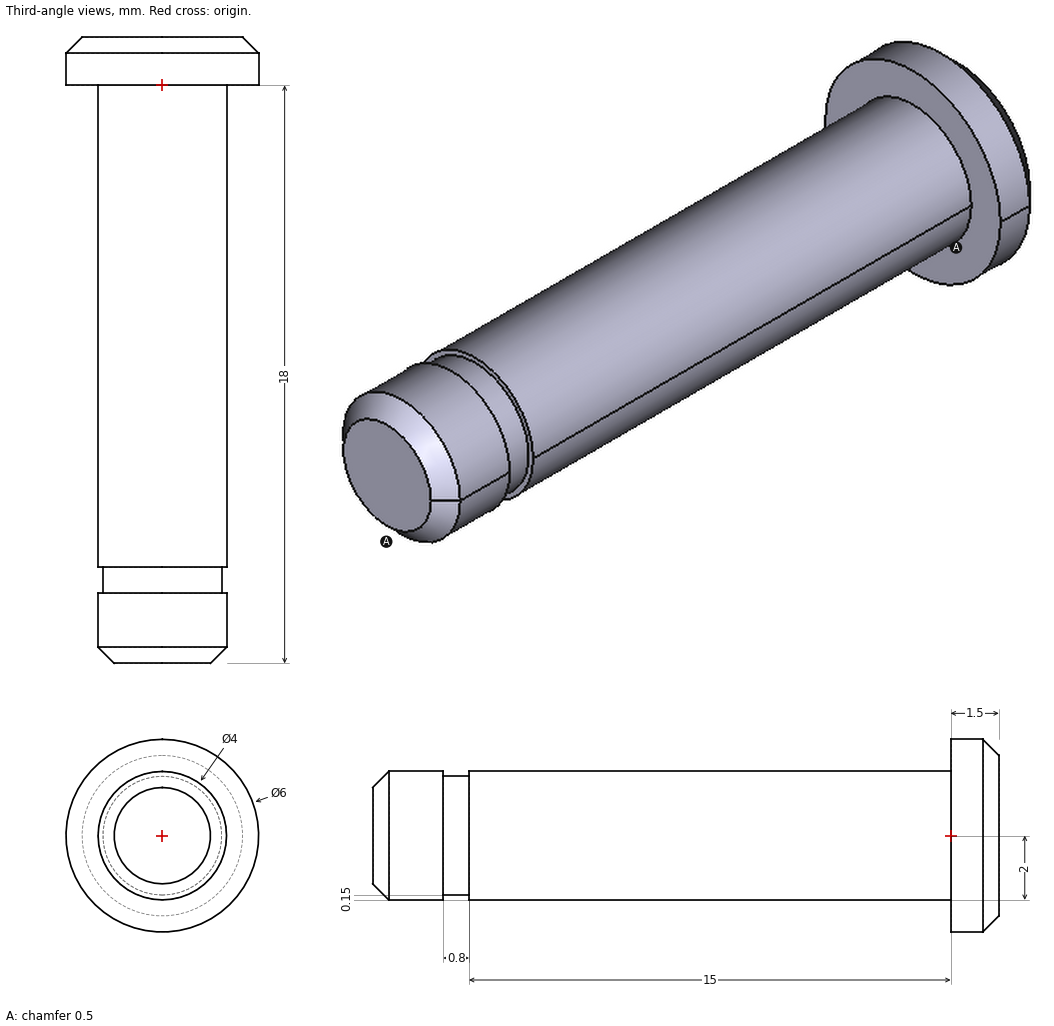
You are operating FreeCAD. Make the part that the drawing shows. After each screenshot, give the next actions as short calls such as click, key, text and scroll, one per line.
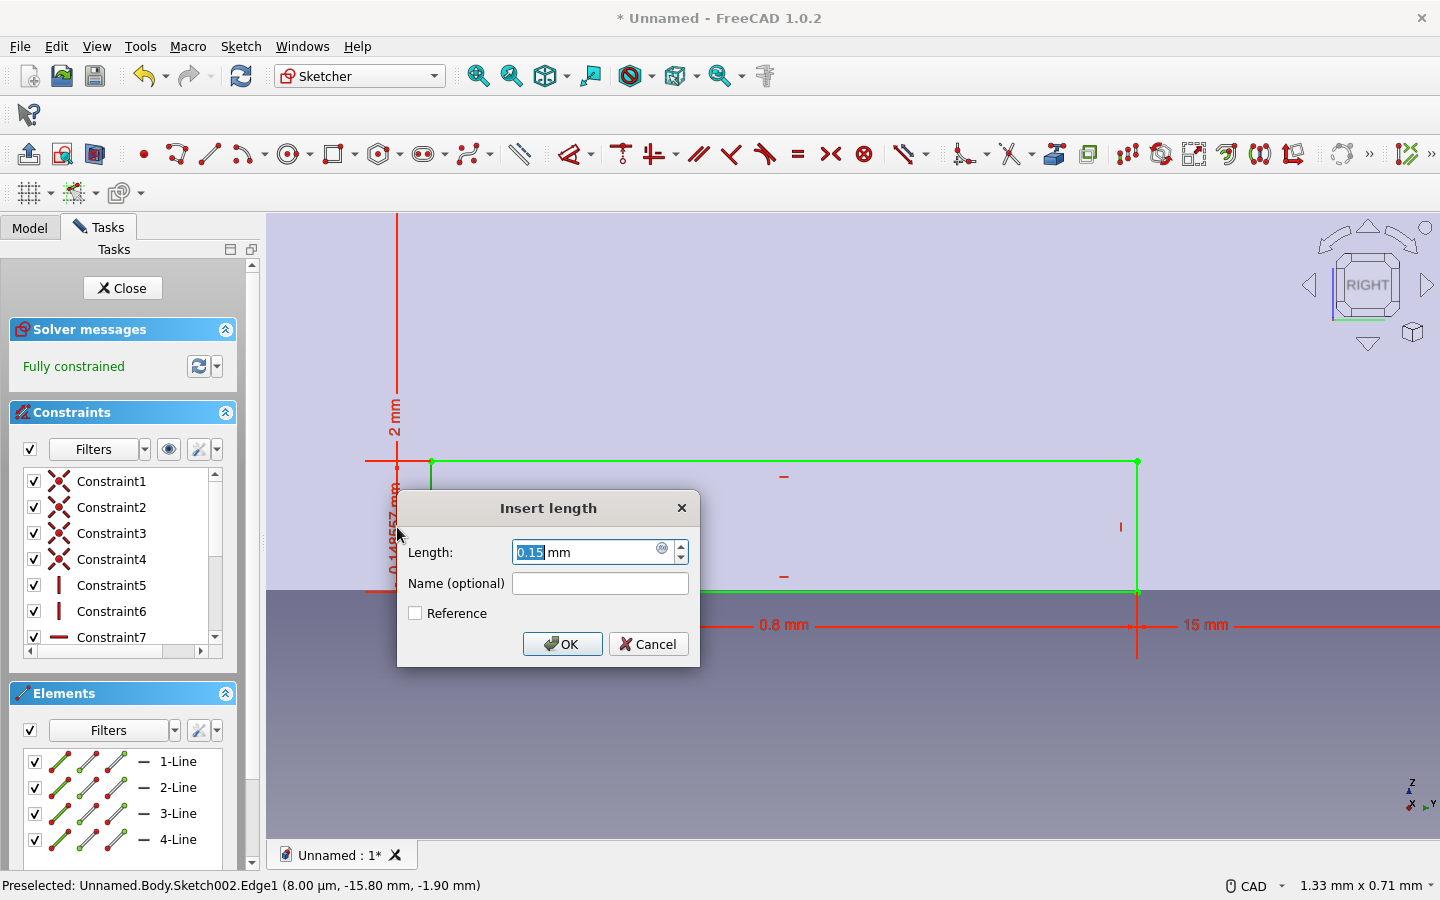
text(0.15)
key(Return)
key(Escape)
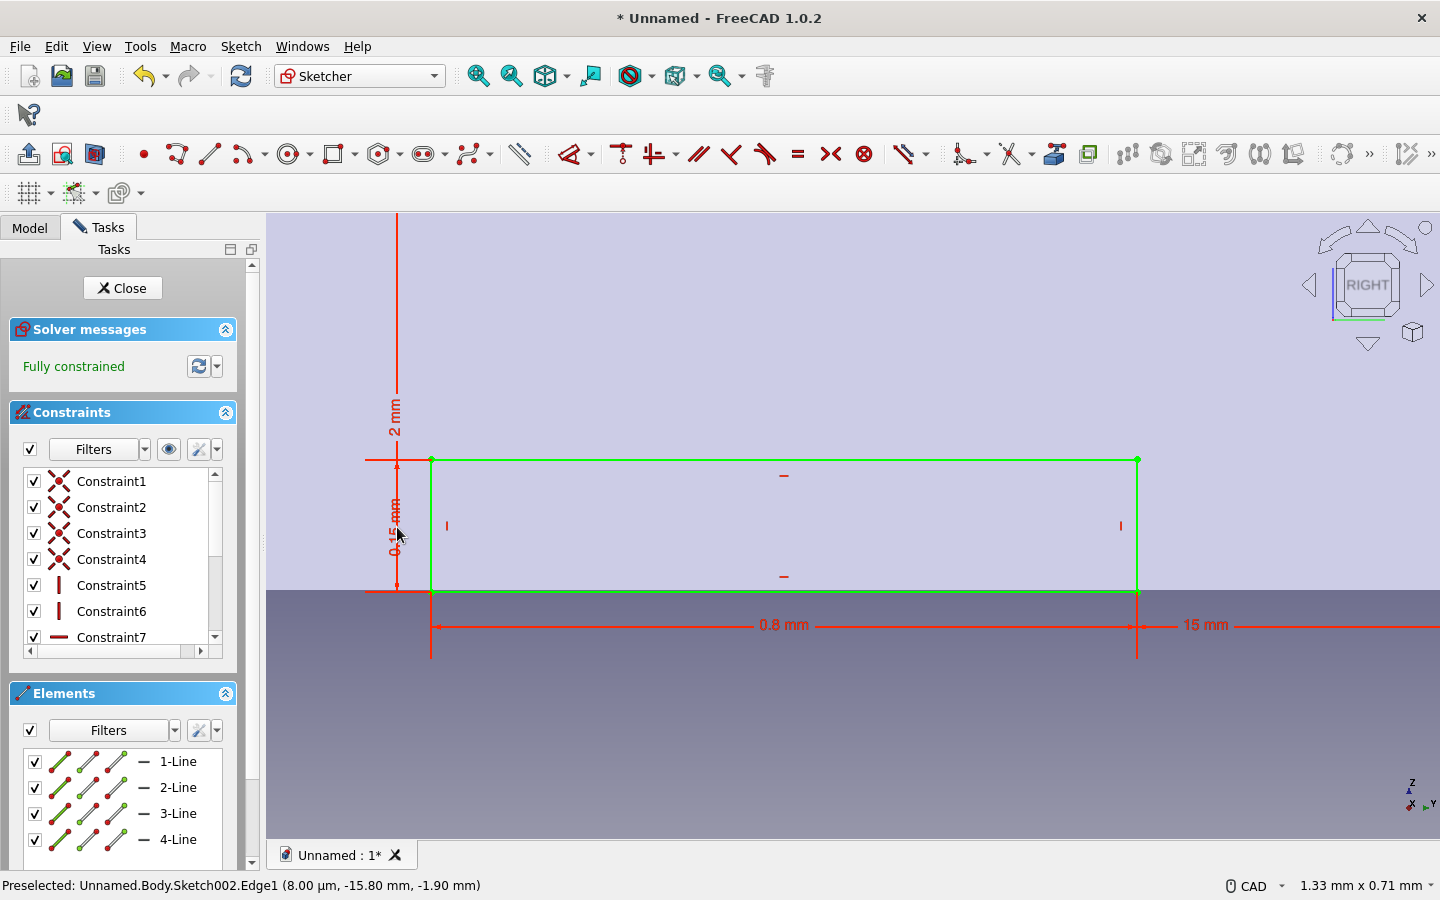
click(123, 288)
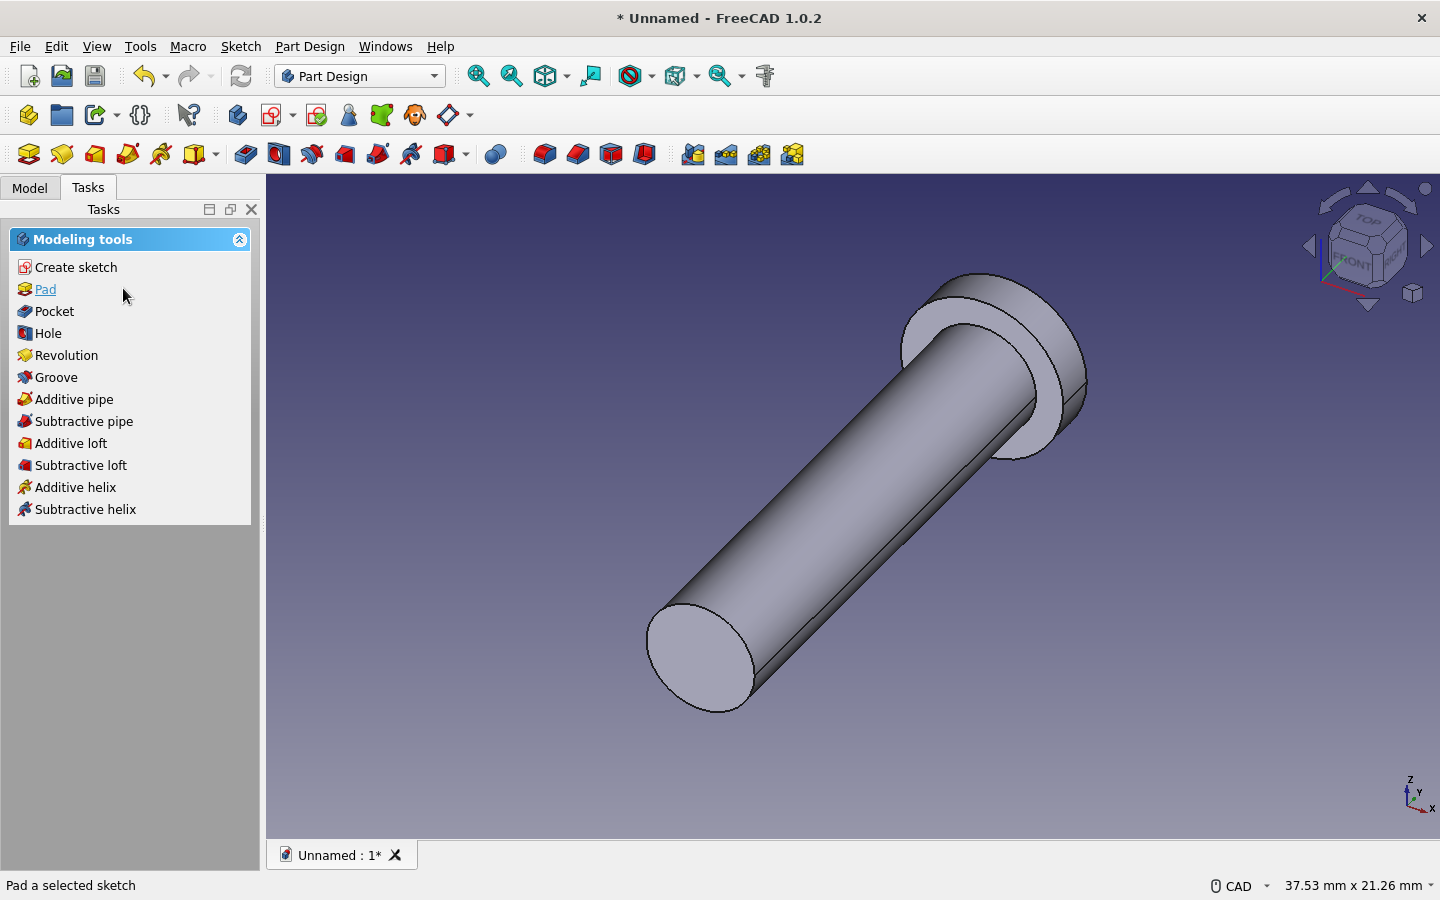
click(312, 154)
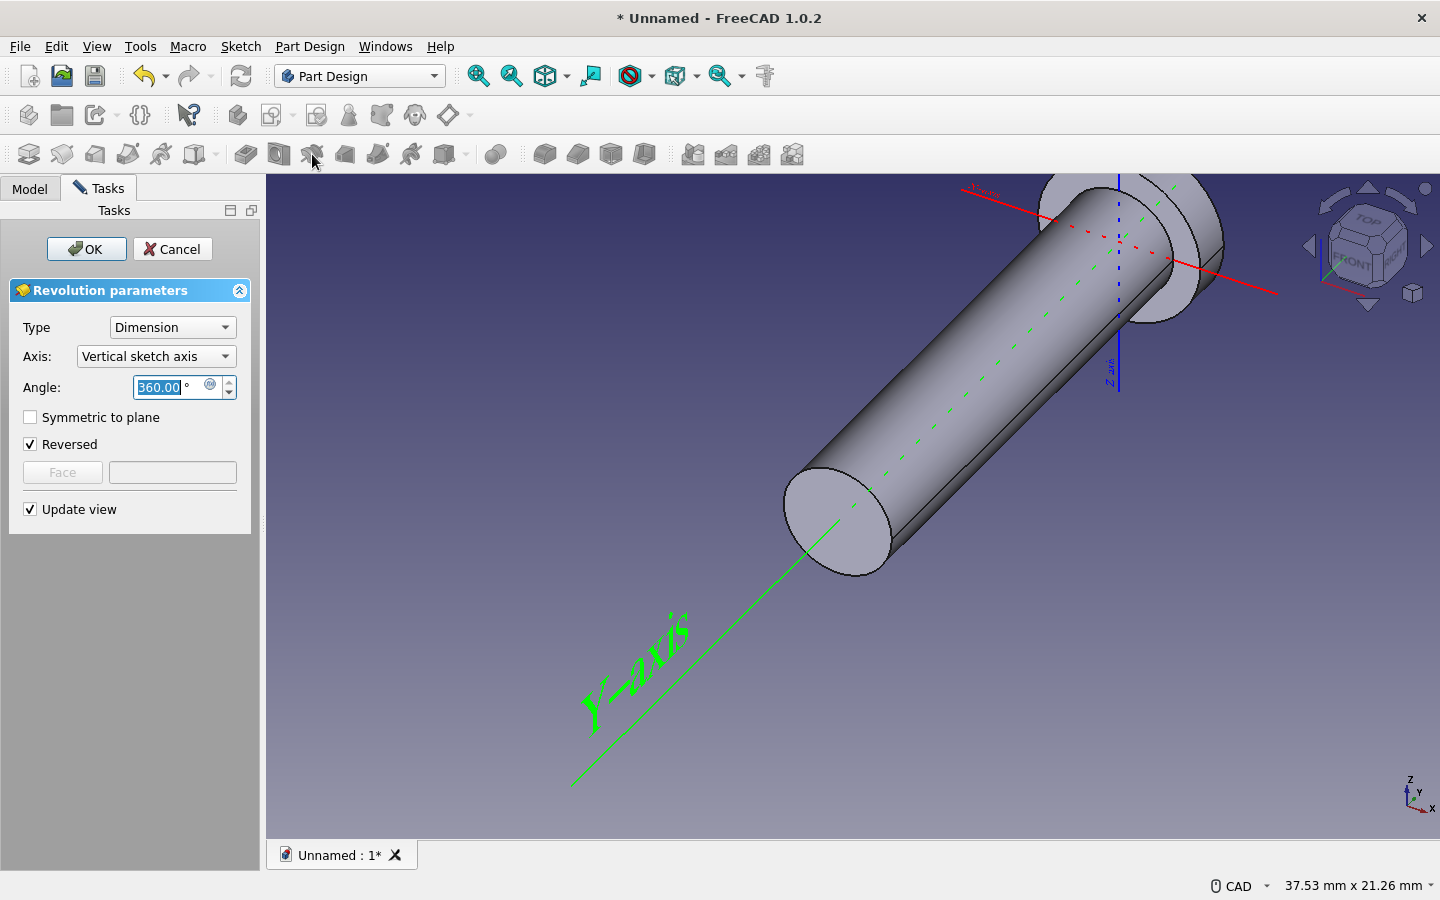
click(157, 356)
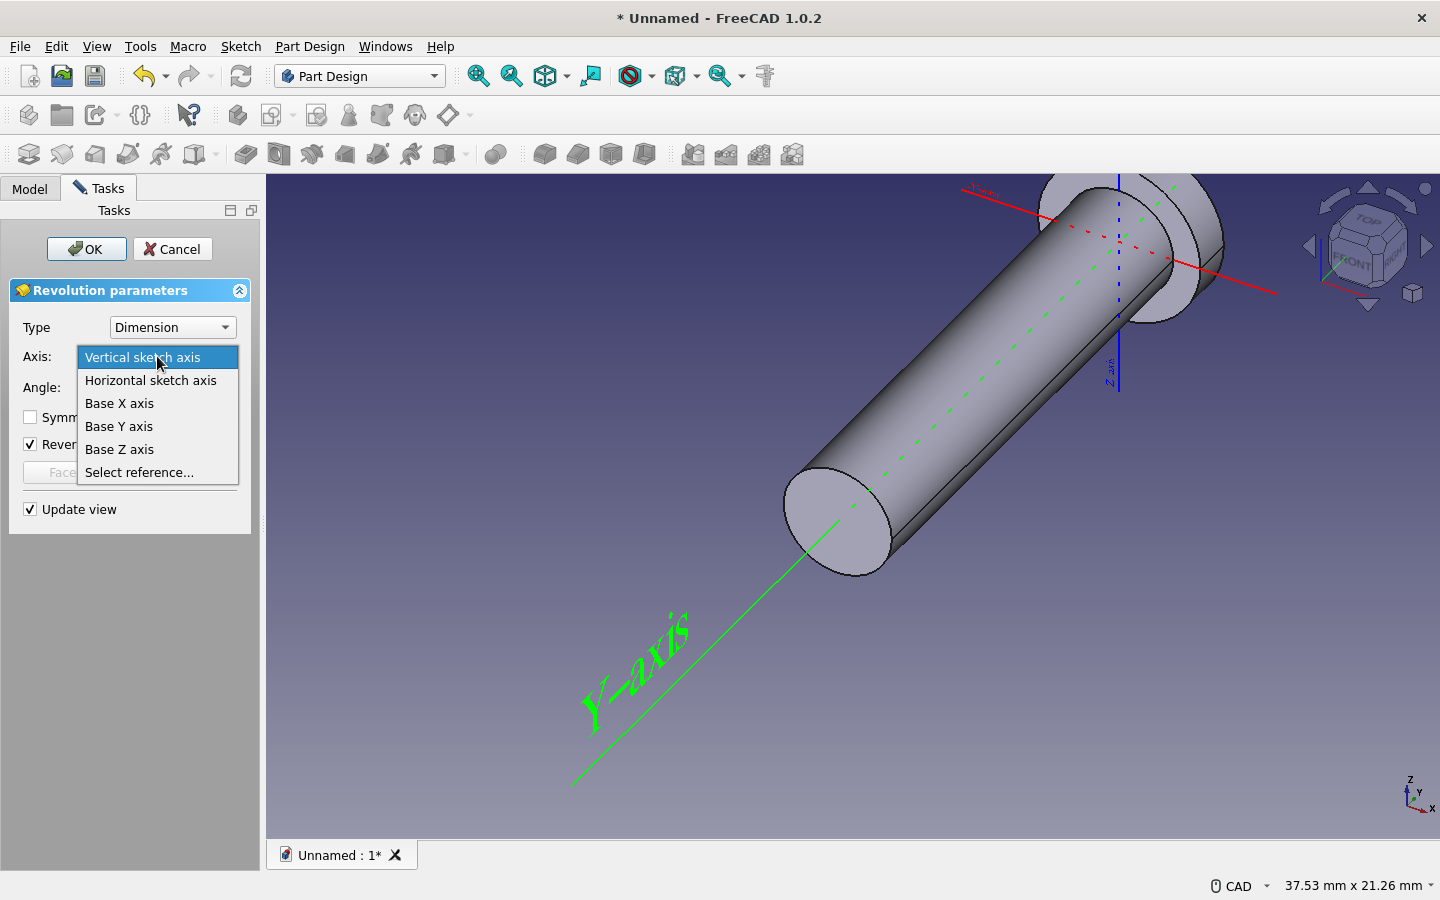
click(156, 380)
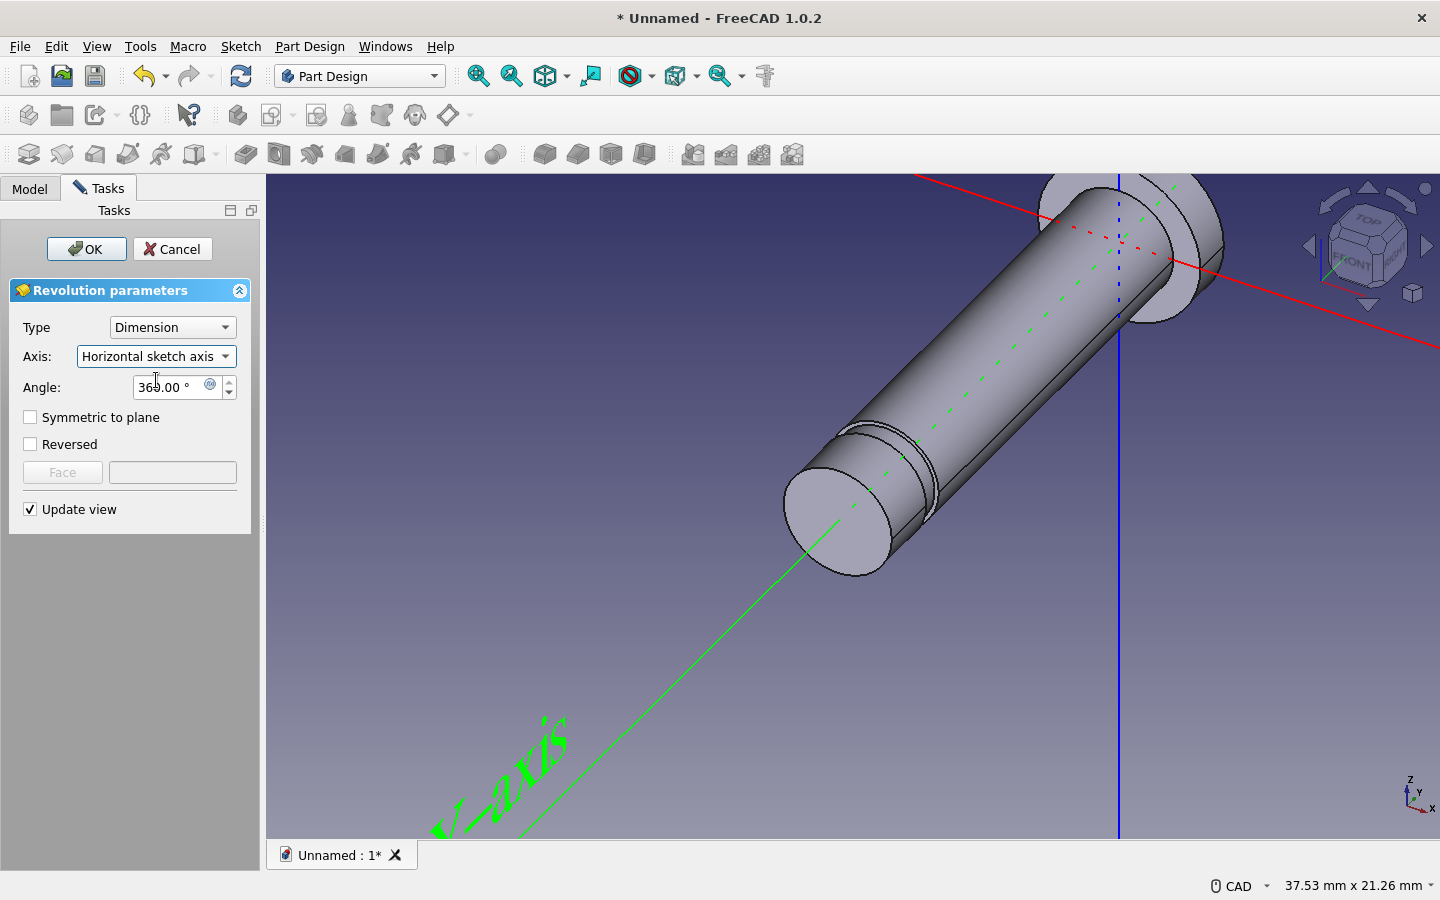
click(87, 249)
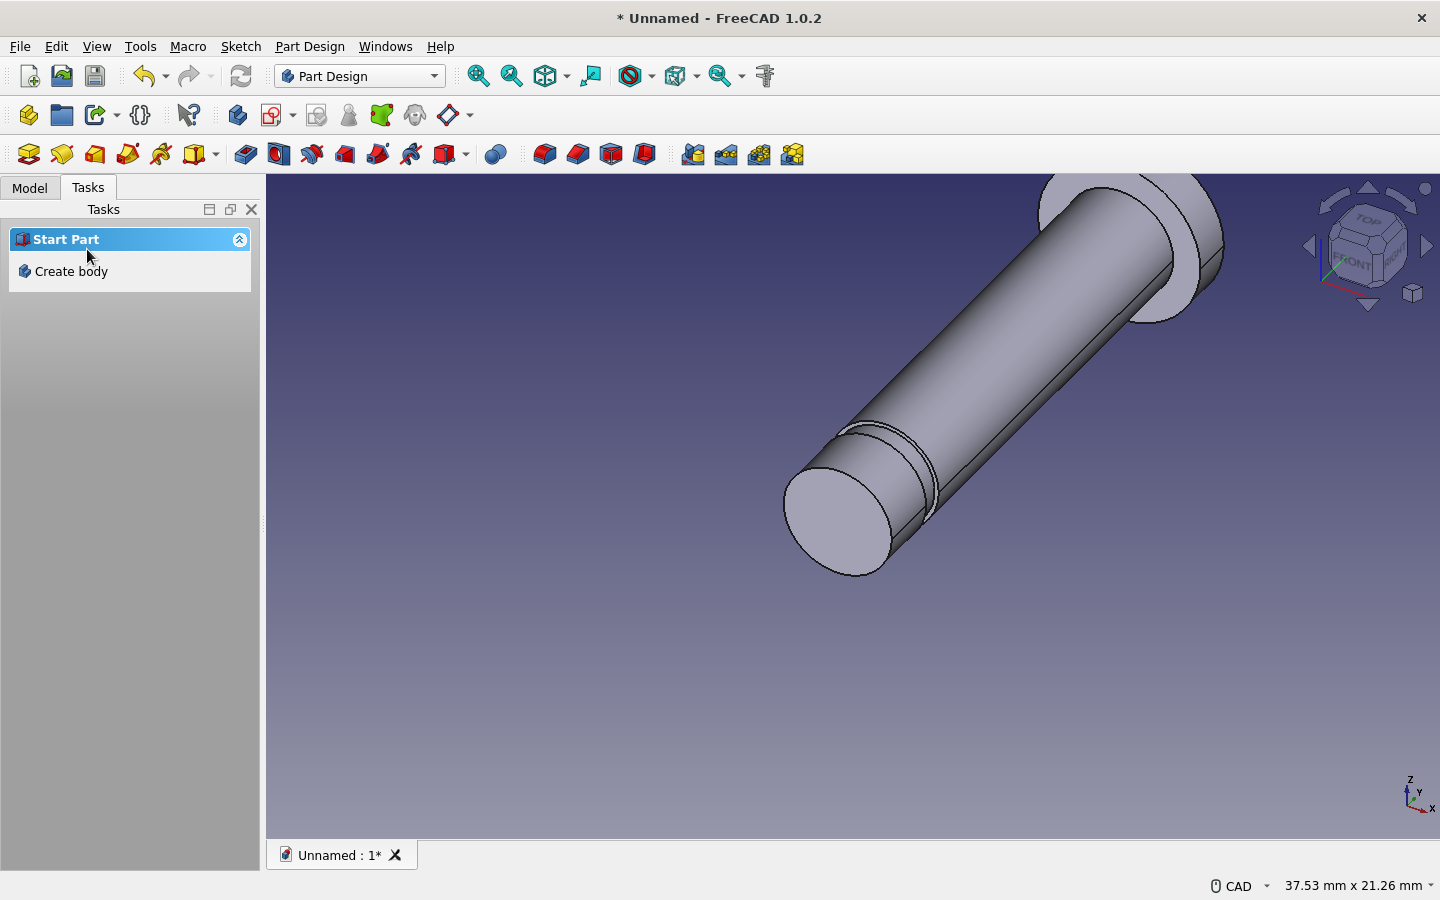
key(v)
key(f)